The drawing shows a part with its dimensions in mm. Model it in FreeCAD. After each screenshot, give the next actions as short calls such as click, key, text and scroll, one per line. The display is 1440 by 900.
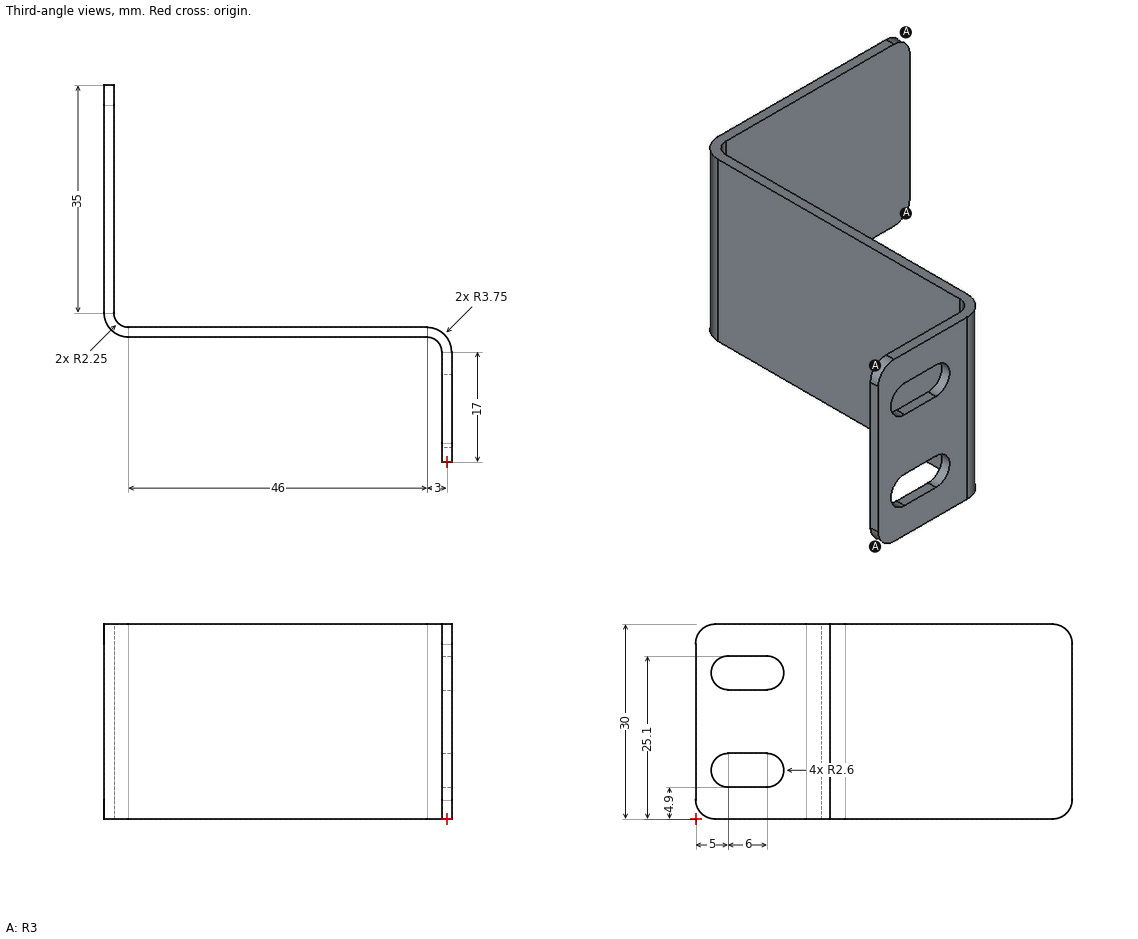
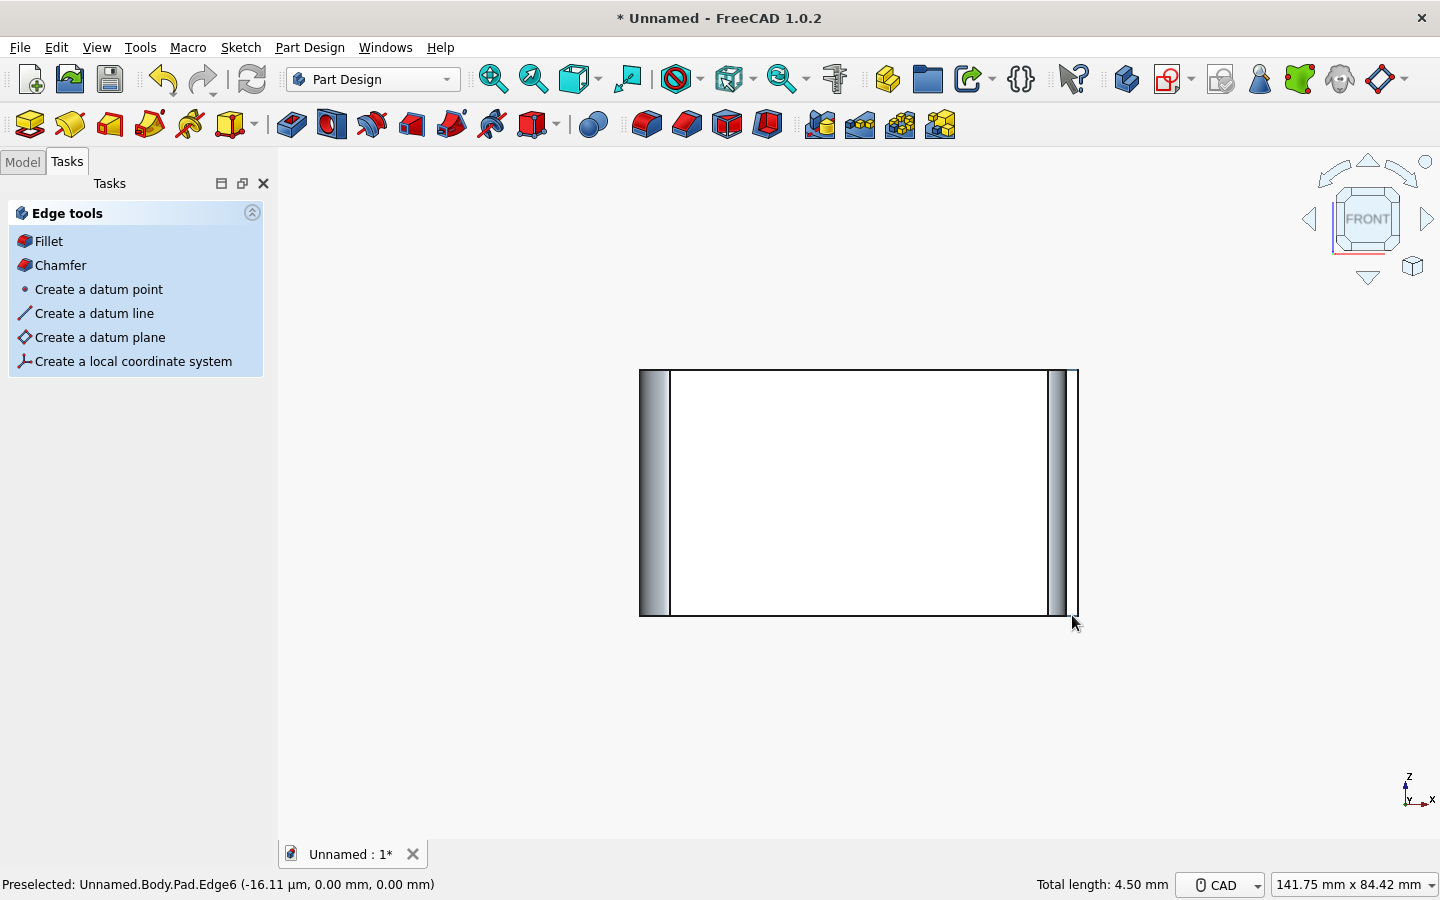
scroll(646, 615, up, 6)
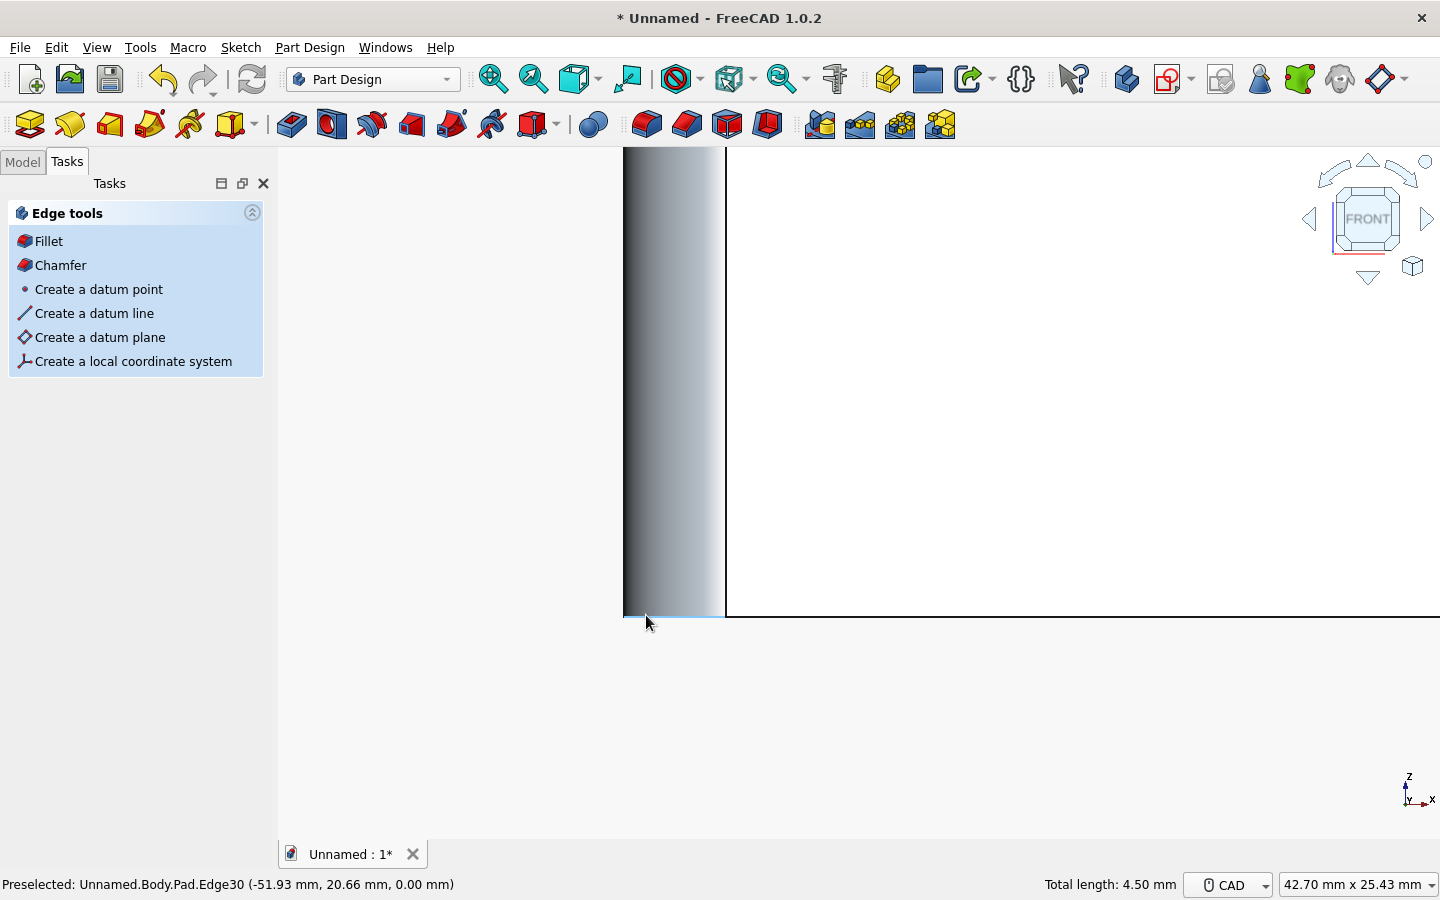
key(v)
key(f)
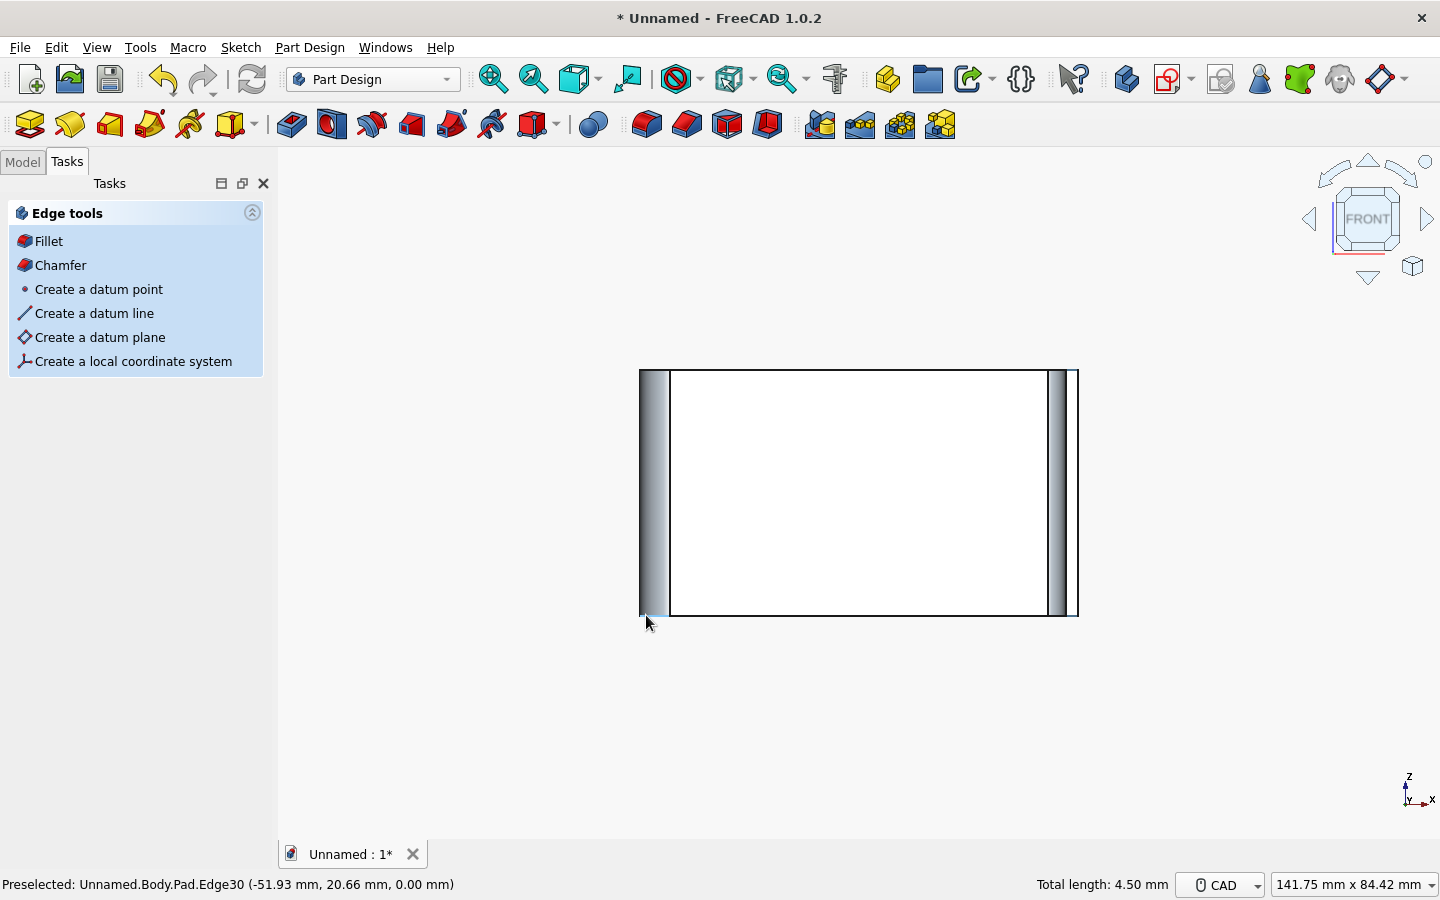
key(3)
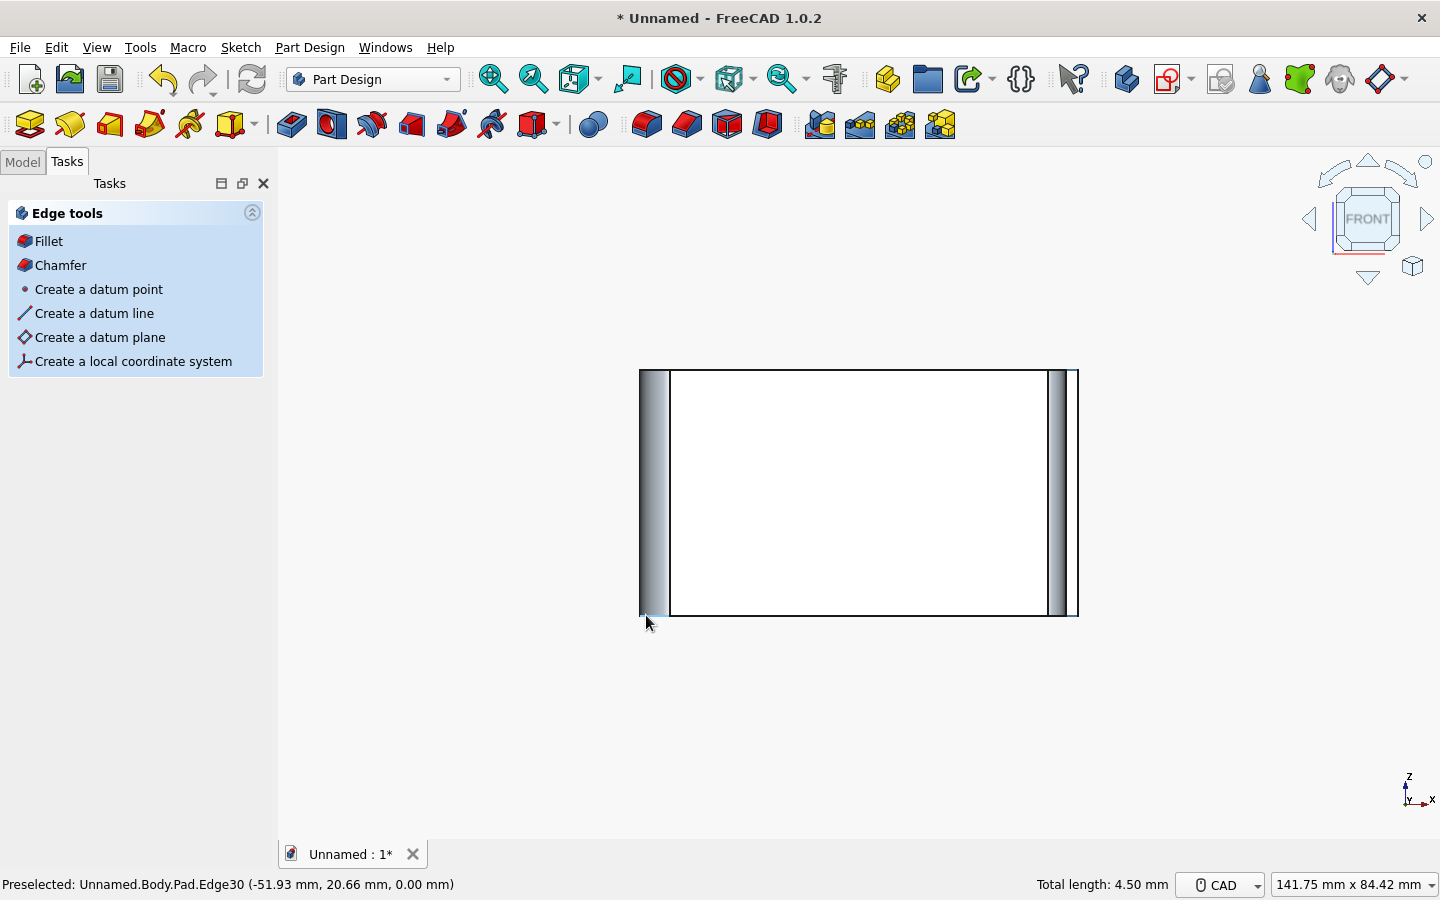
key(v)
key(f)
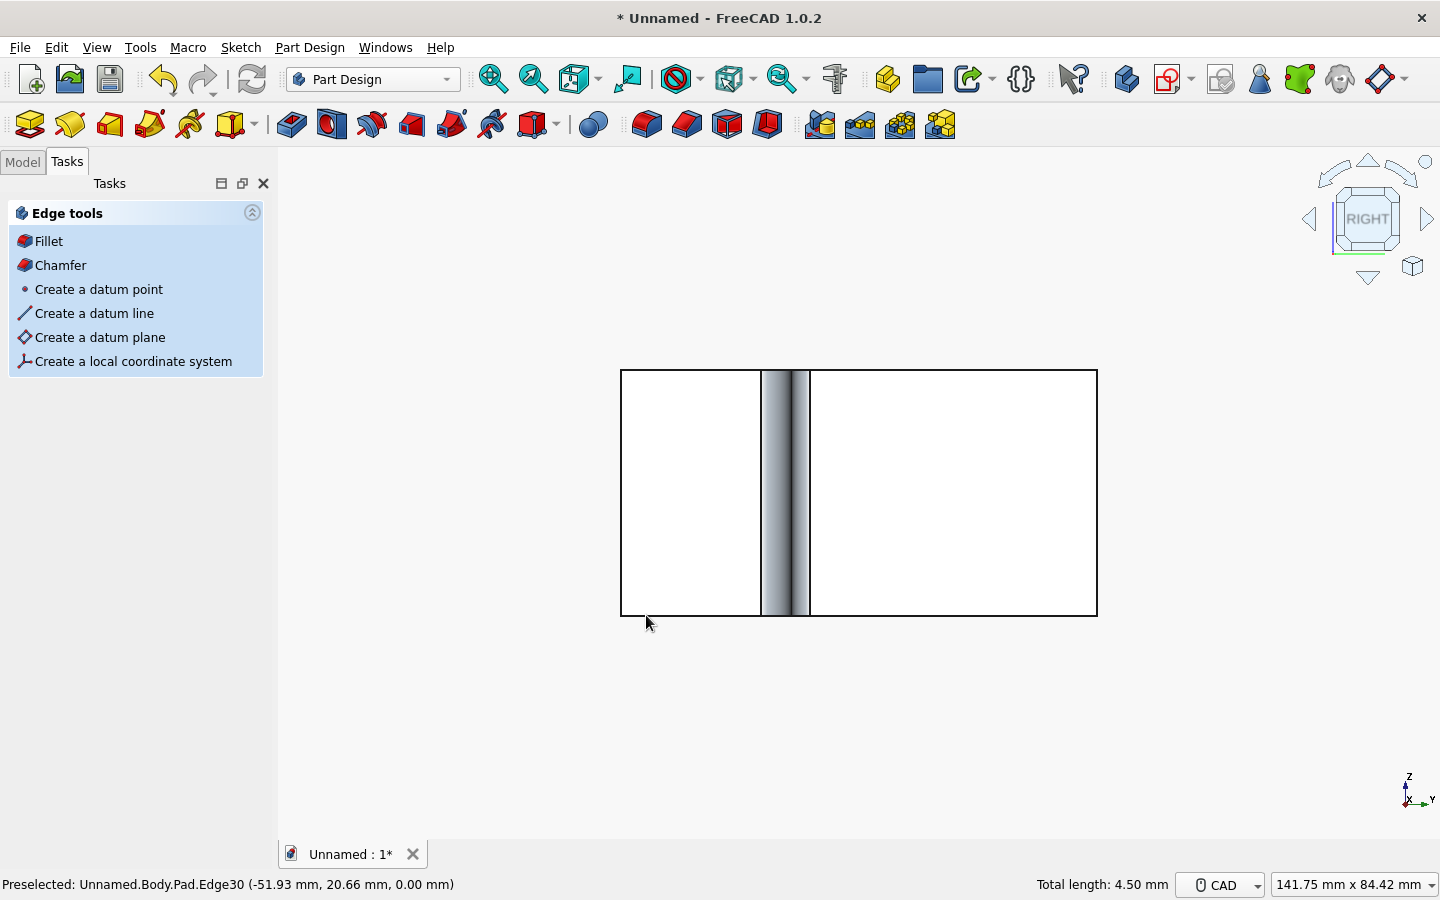
scroll(1097, 615, up, 6)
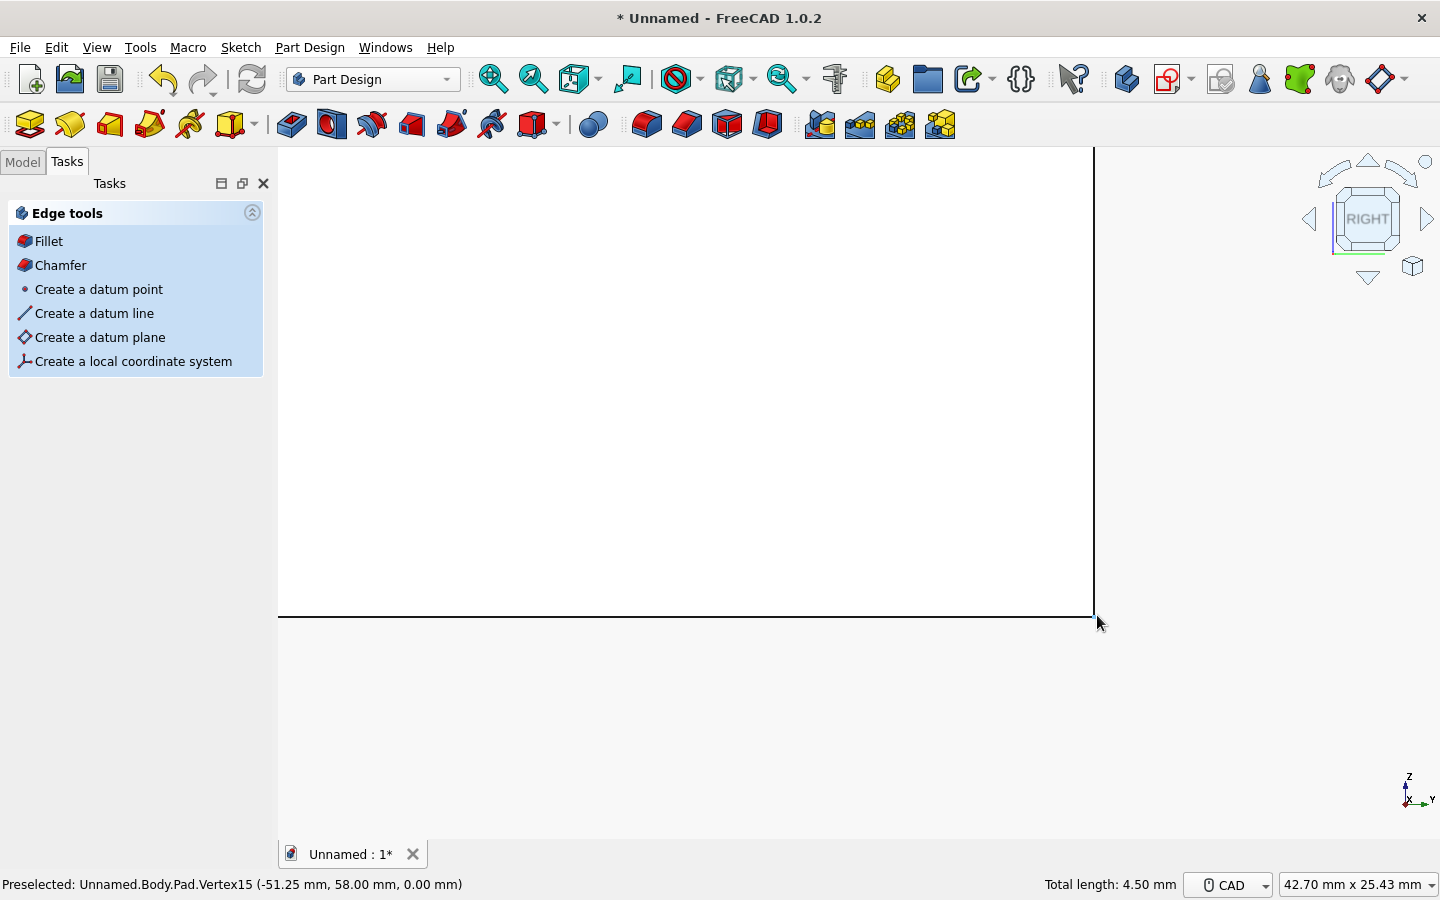
click(494, 80)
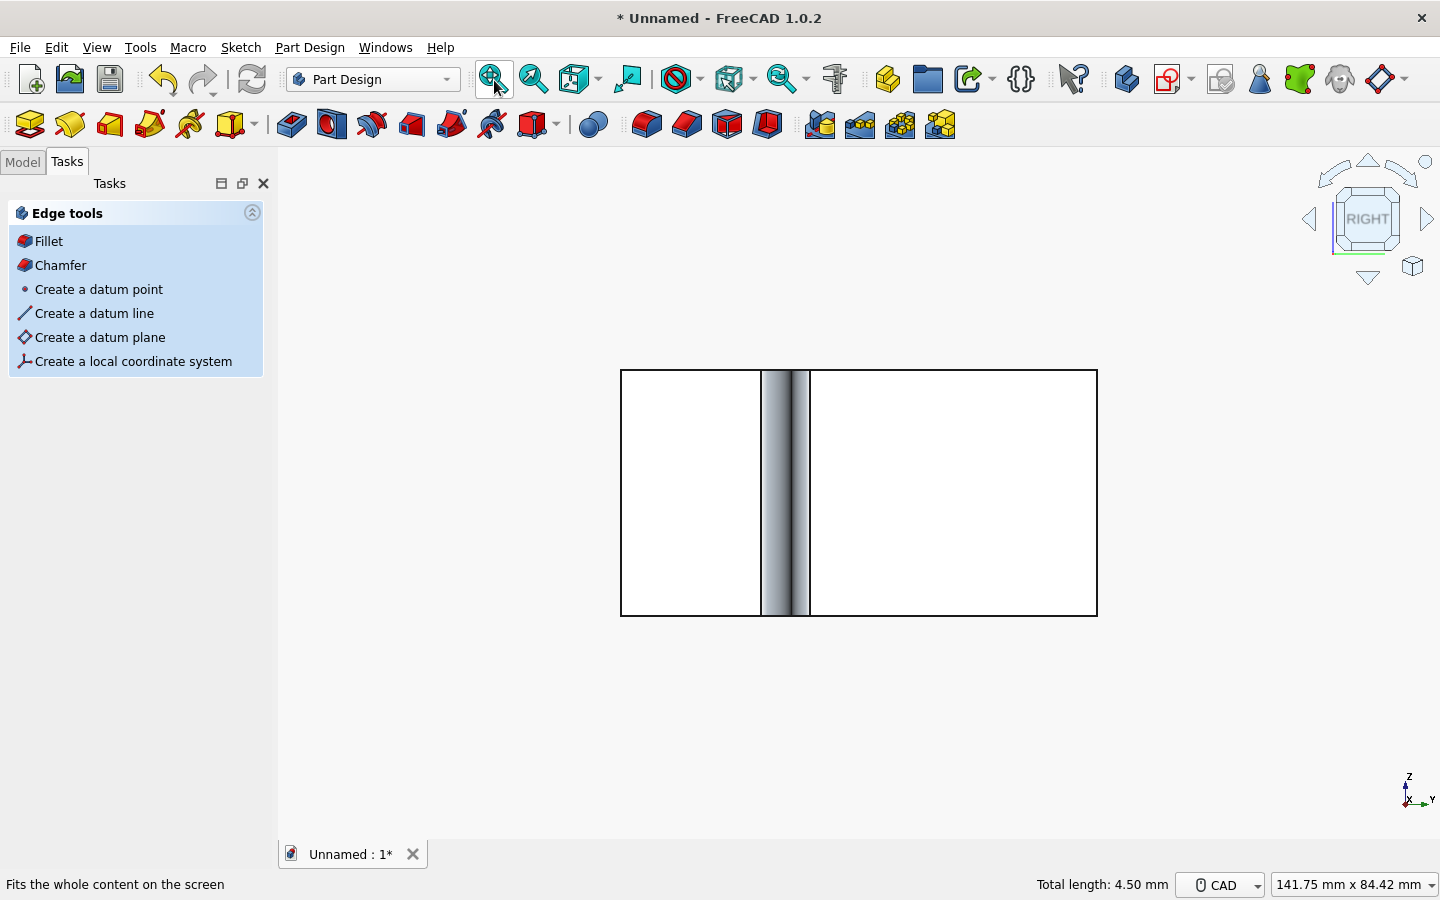
key(5)